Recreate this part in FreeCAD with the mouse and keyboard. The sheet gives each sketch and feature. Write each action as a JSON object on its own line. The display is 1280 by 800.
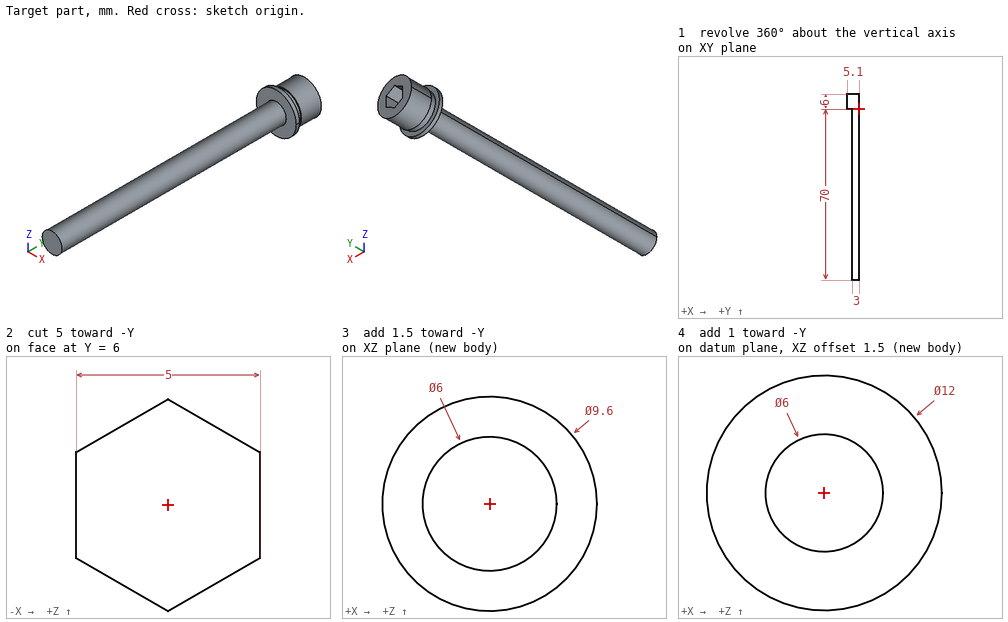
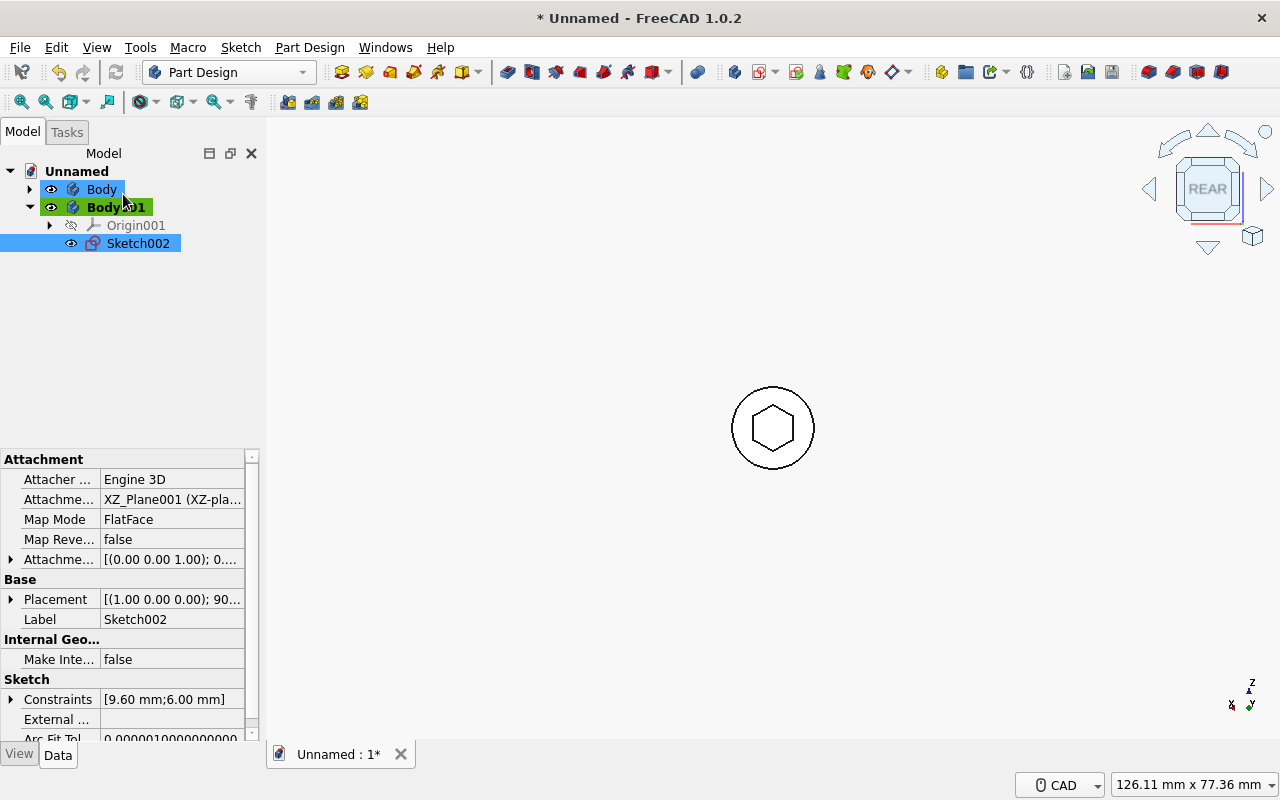
{"action": "left_click", "coordinate": [342, 72]}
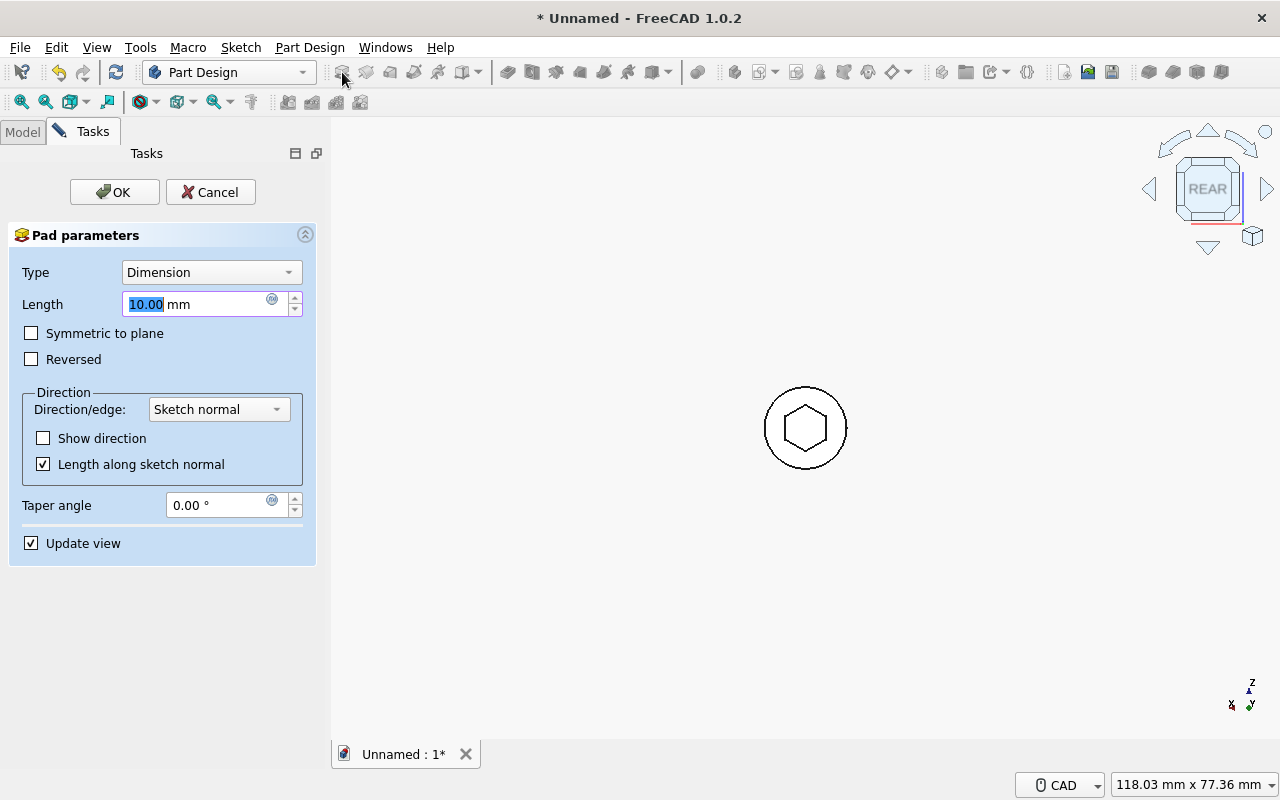
{"action": "type", "text": "1.5"}
{"action": "key", "text": "Tab"}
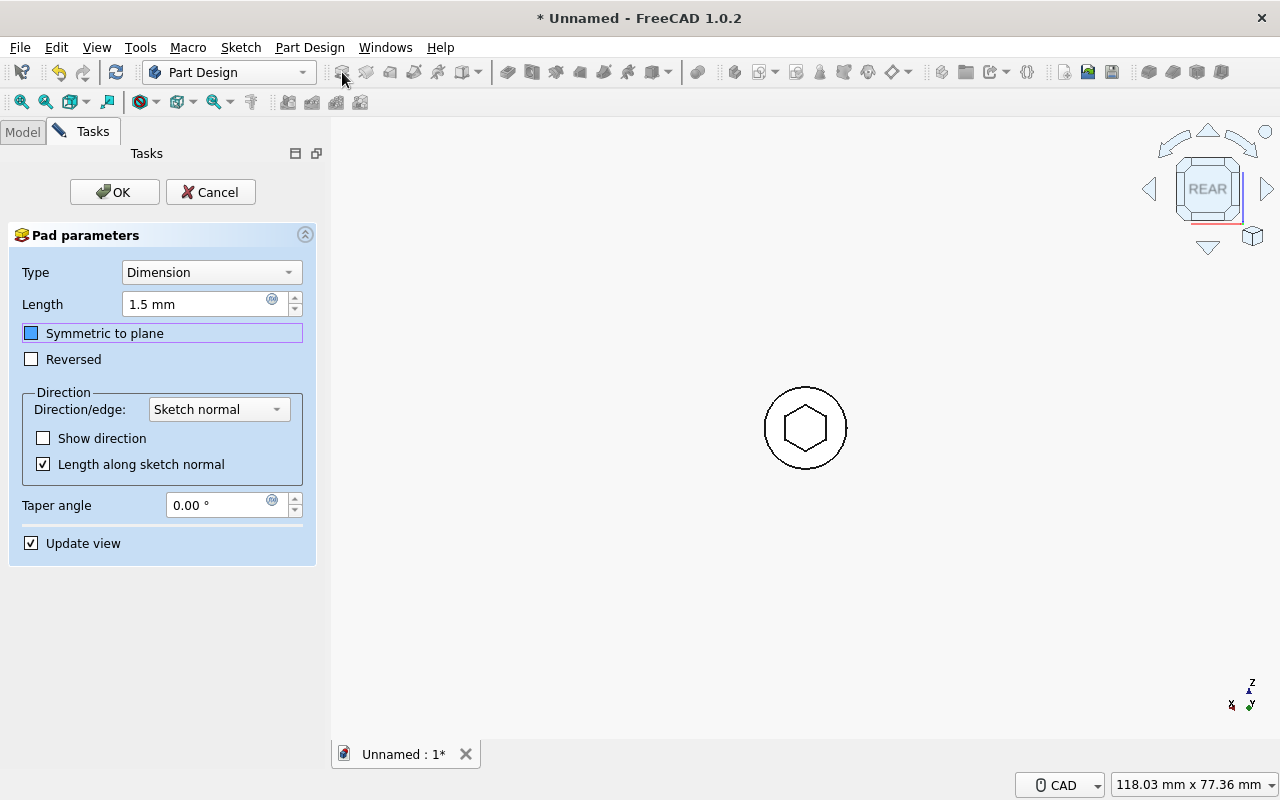
{"action": "left_click", "coordinate": [115, 192]}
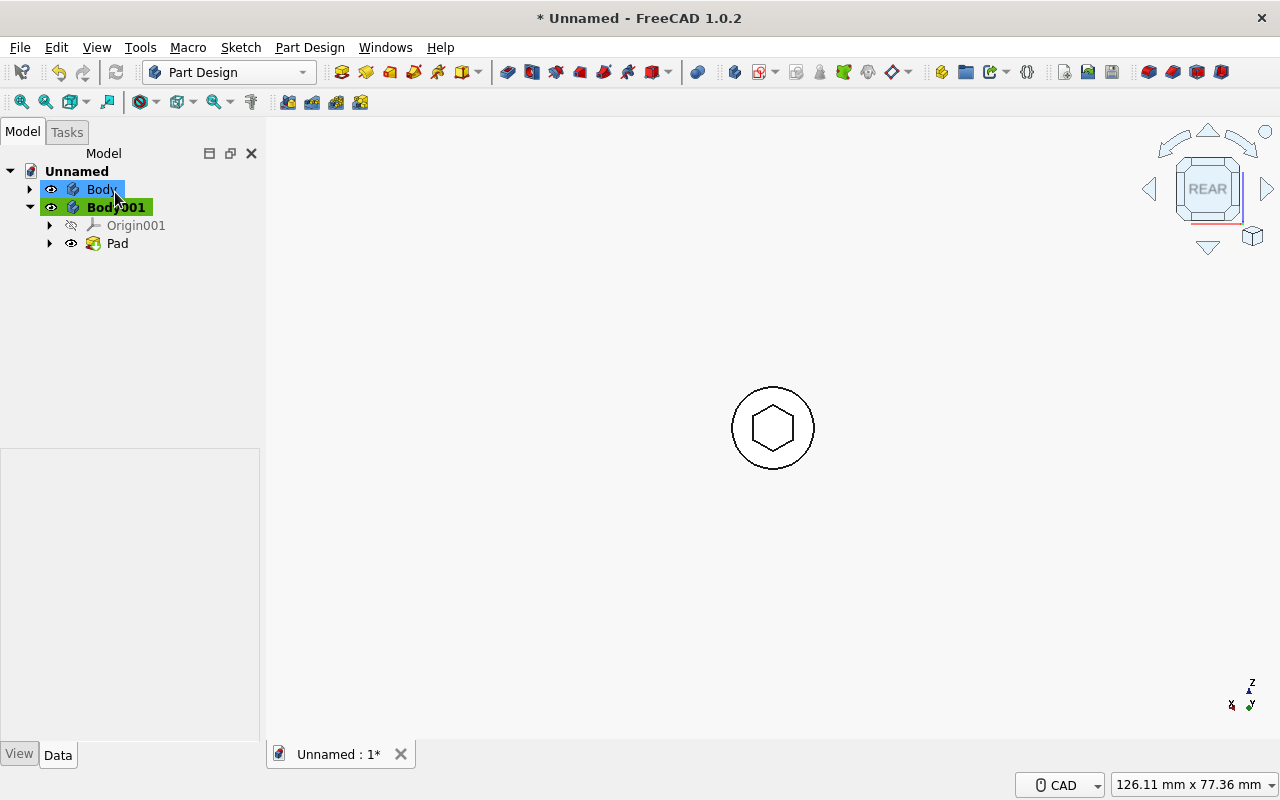
{"action": "key", "text": "v f"}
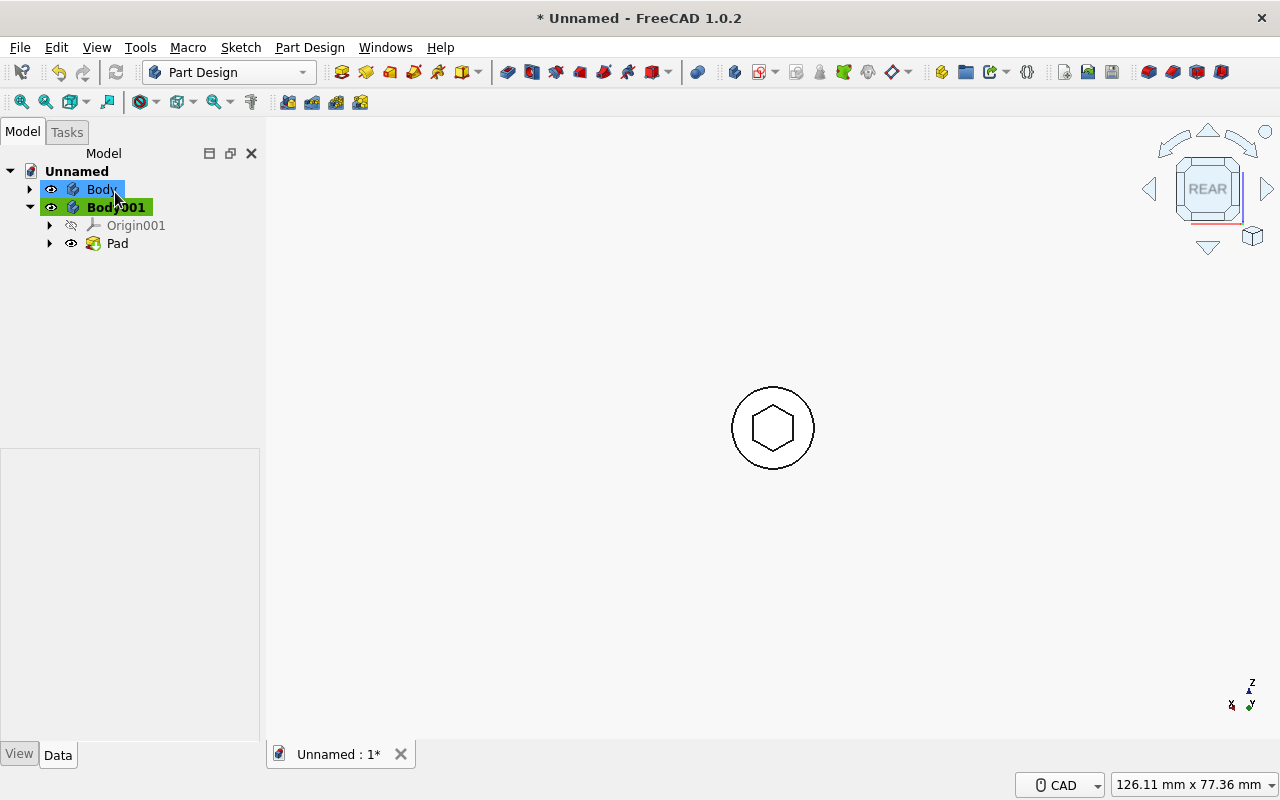
{"action": "left_click", "coordinate": [736, 72]}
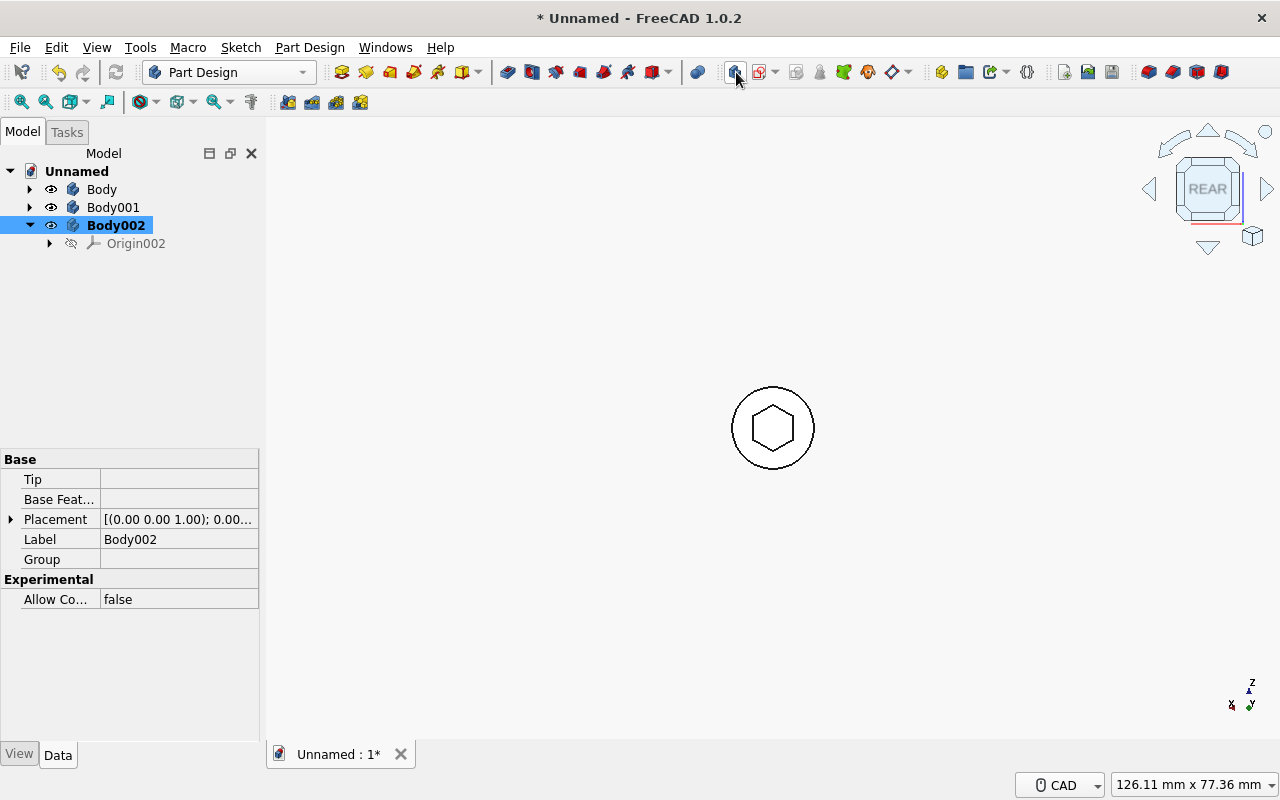
{"action": "left_click", "coordinate": [50, 243]}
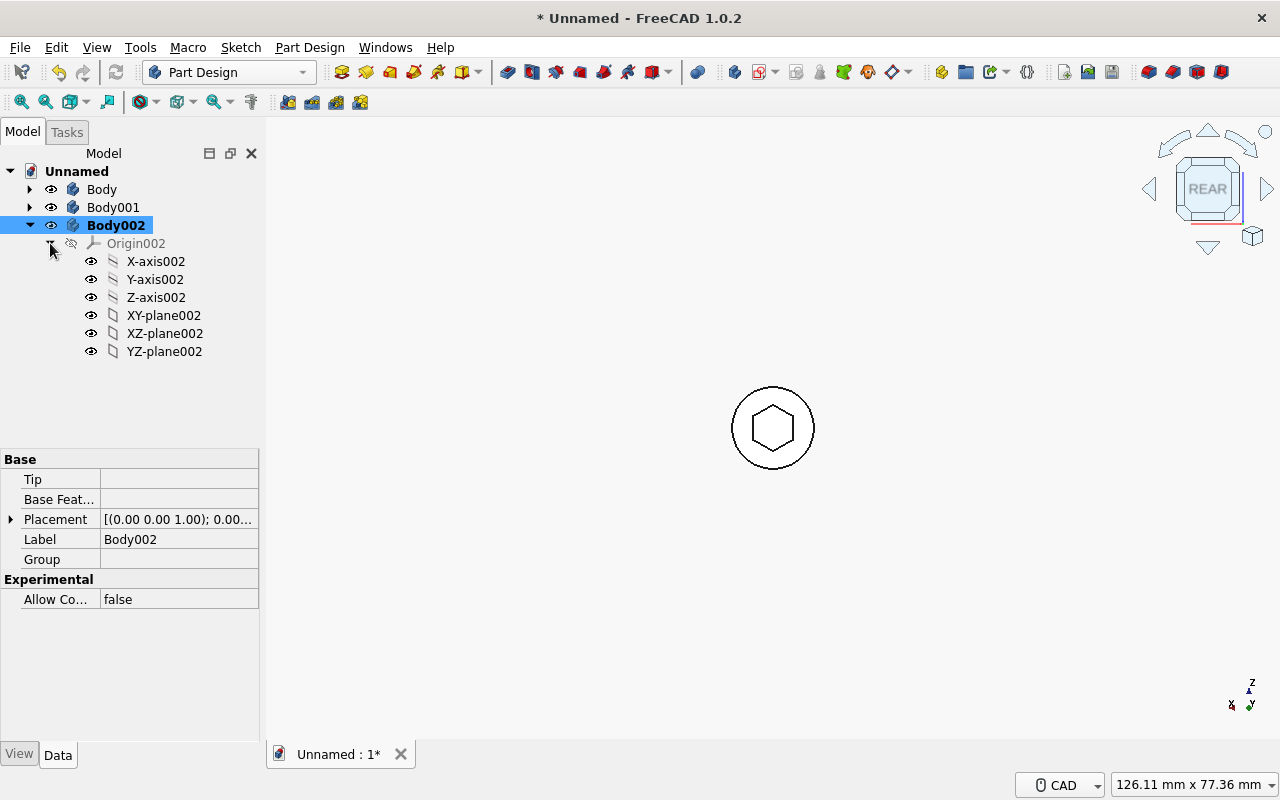
{"action": "left_click", "coordinate": [136, 333]}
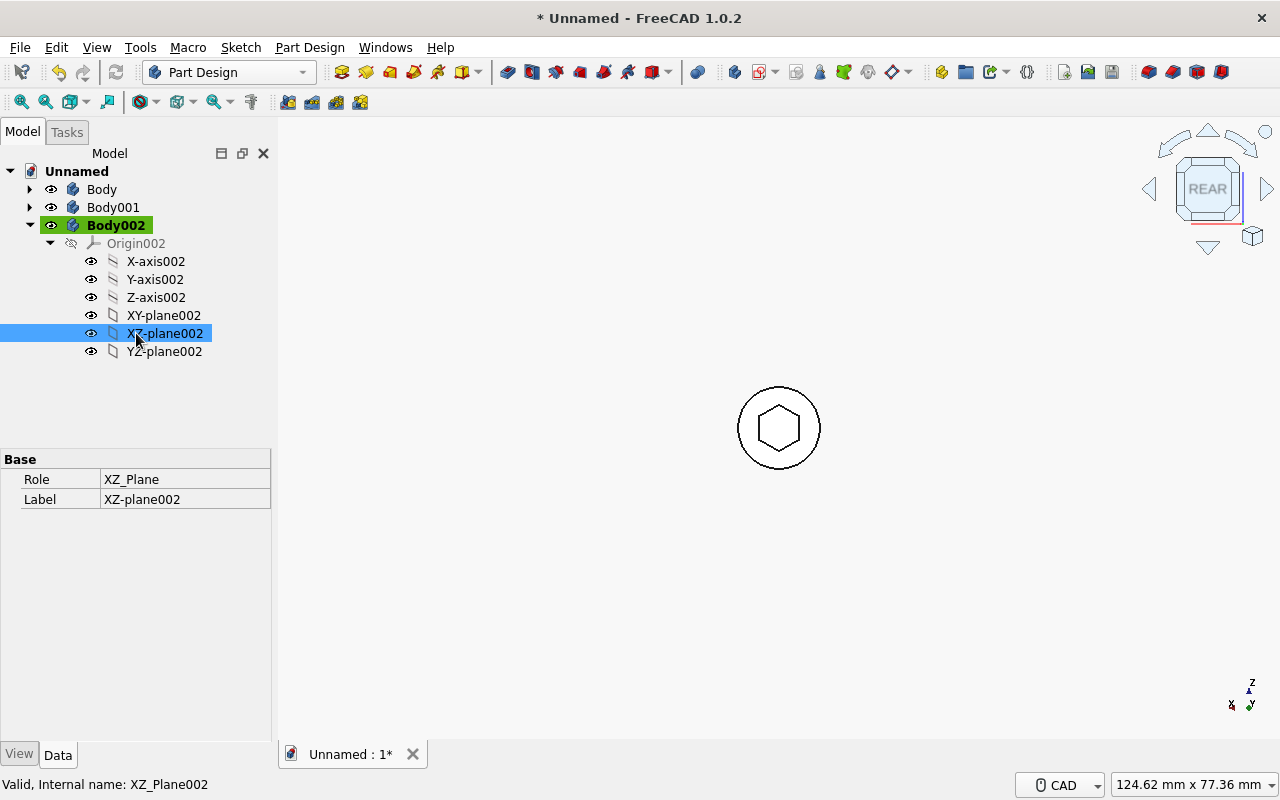
{"action": "left_click", "coordinate": [892, 72]}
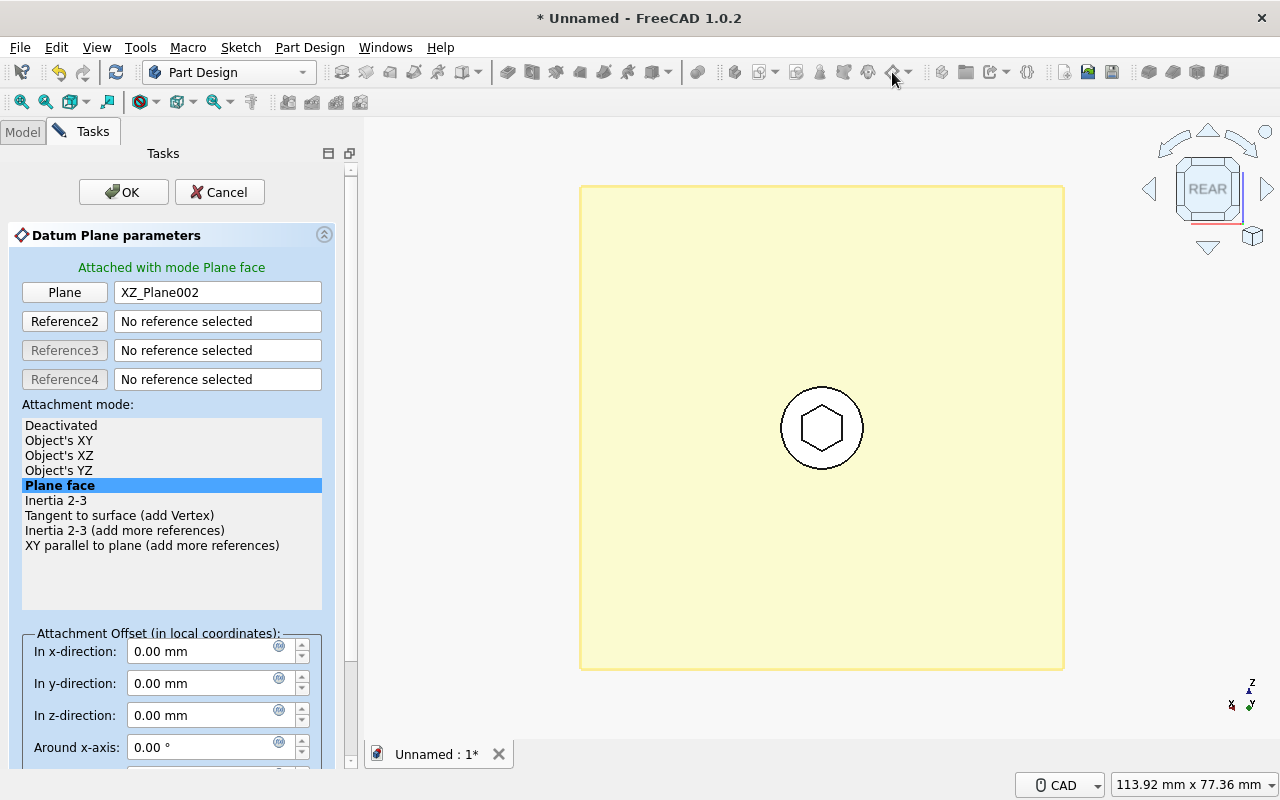
{"action": "triple_click", "coordinate": [210, 715]}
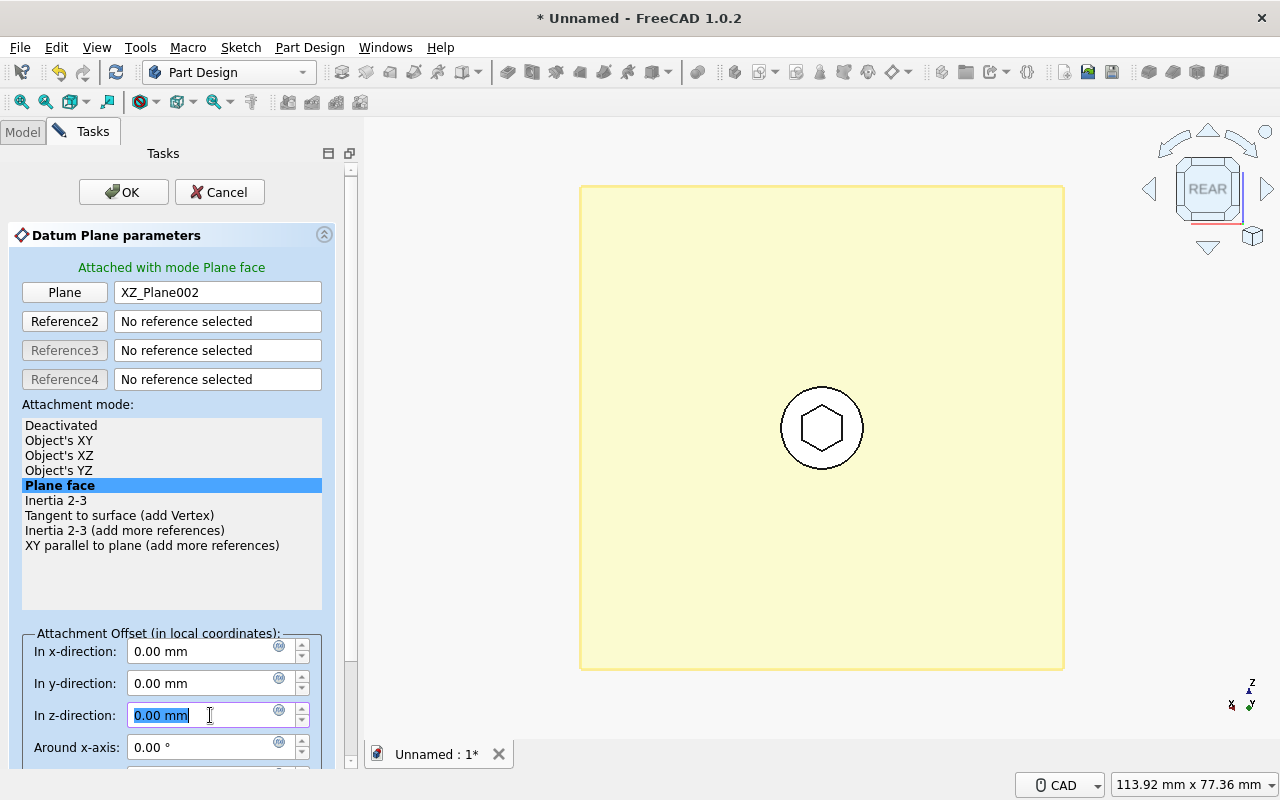
{"action": "type", "text": "1.5"}
{"action": "key", "text": "Tab"}